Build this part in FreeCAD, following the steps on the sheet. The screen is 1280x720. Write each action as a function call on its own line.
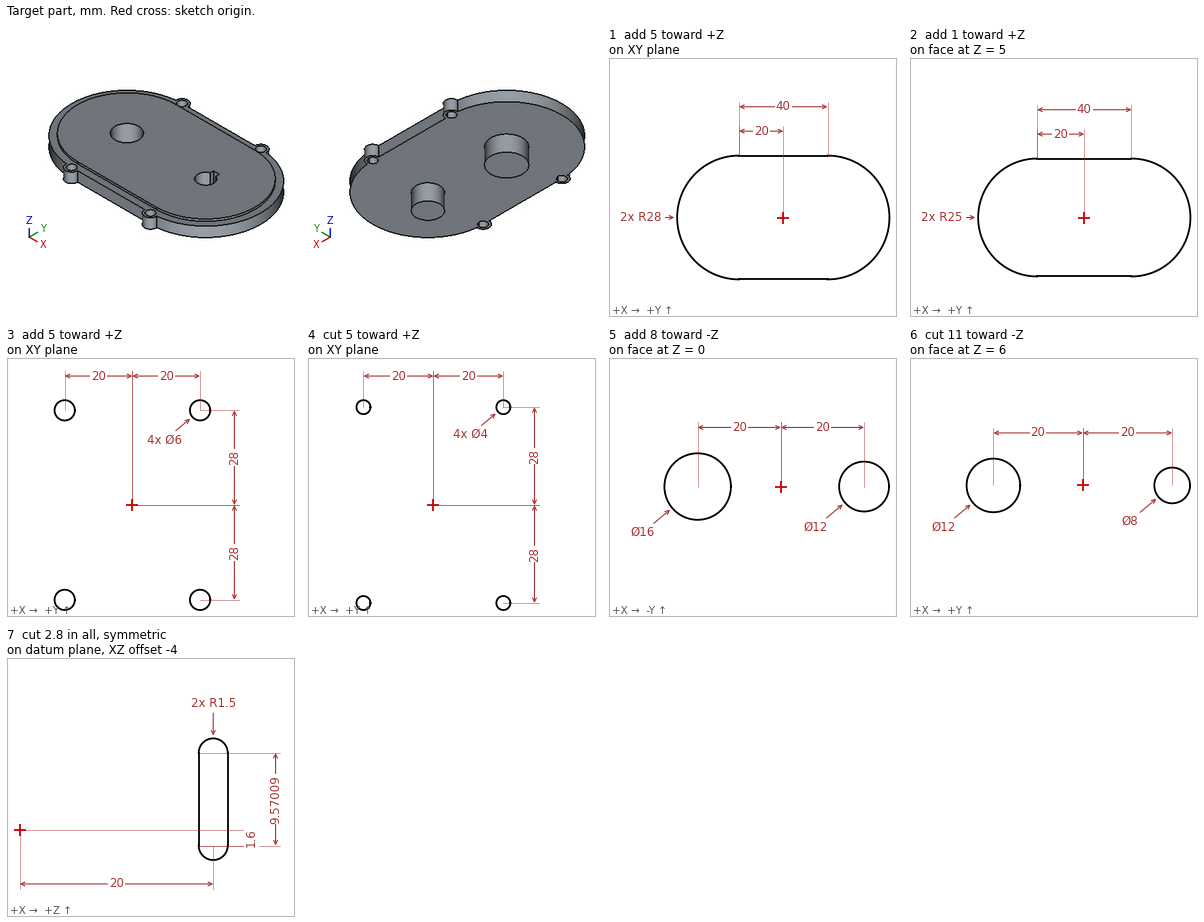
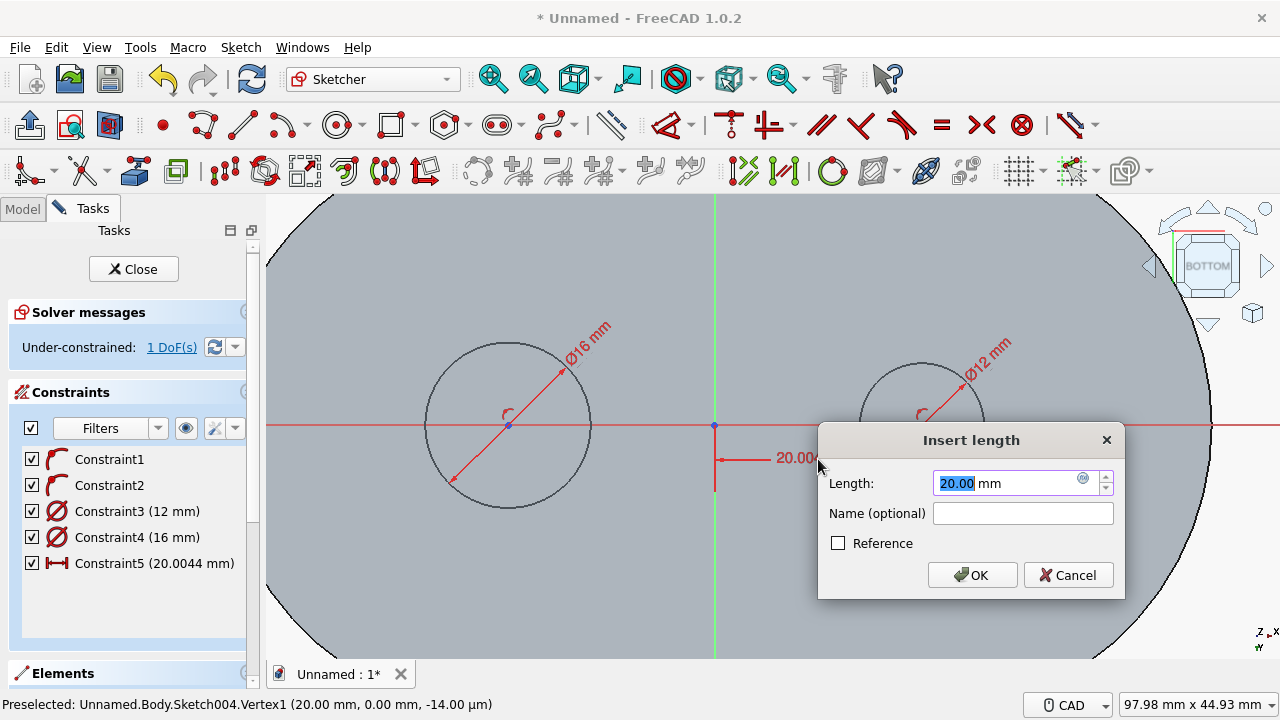
text(20)
key(Return)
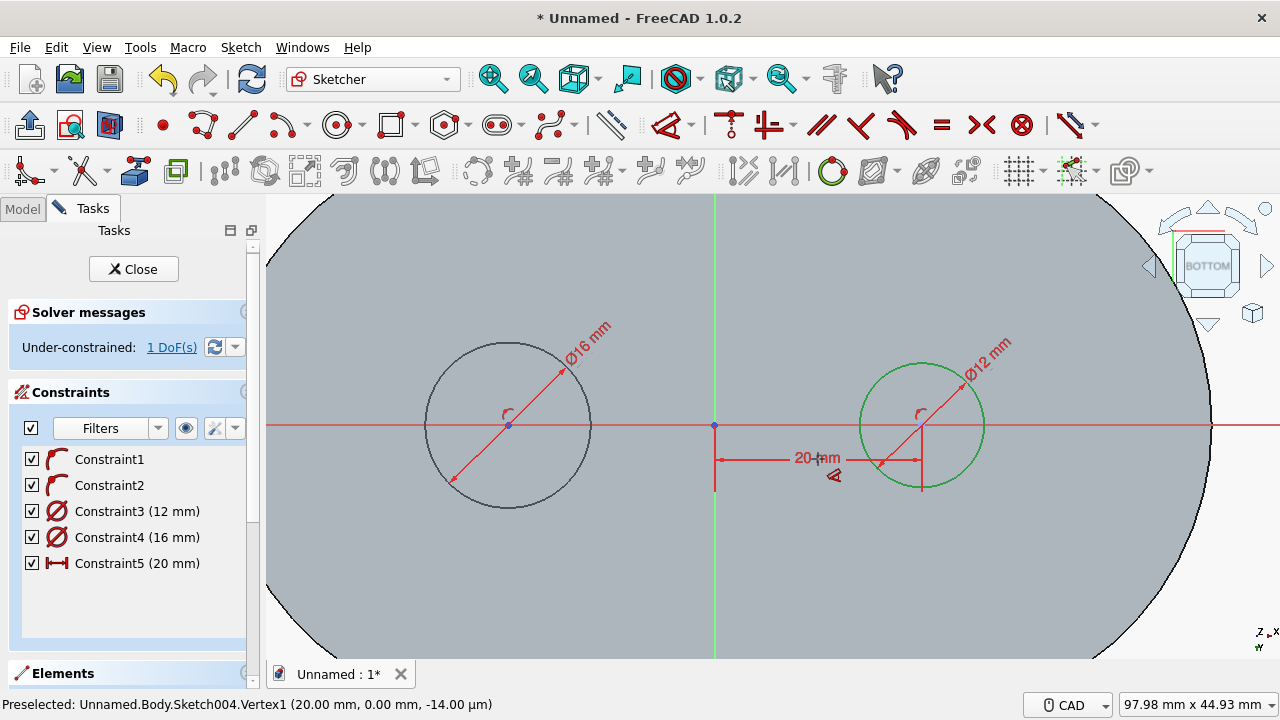
click(508, 425)
click(611, 459)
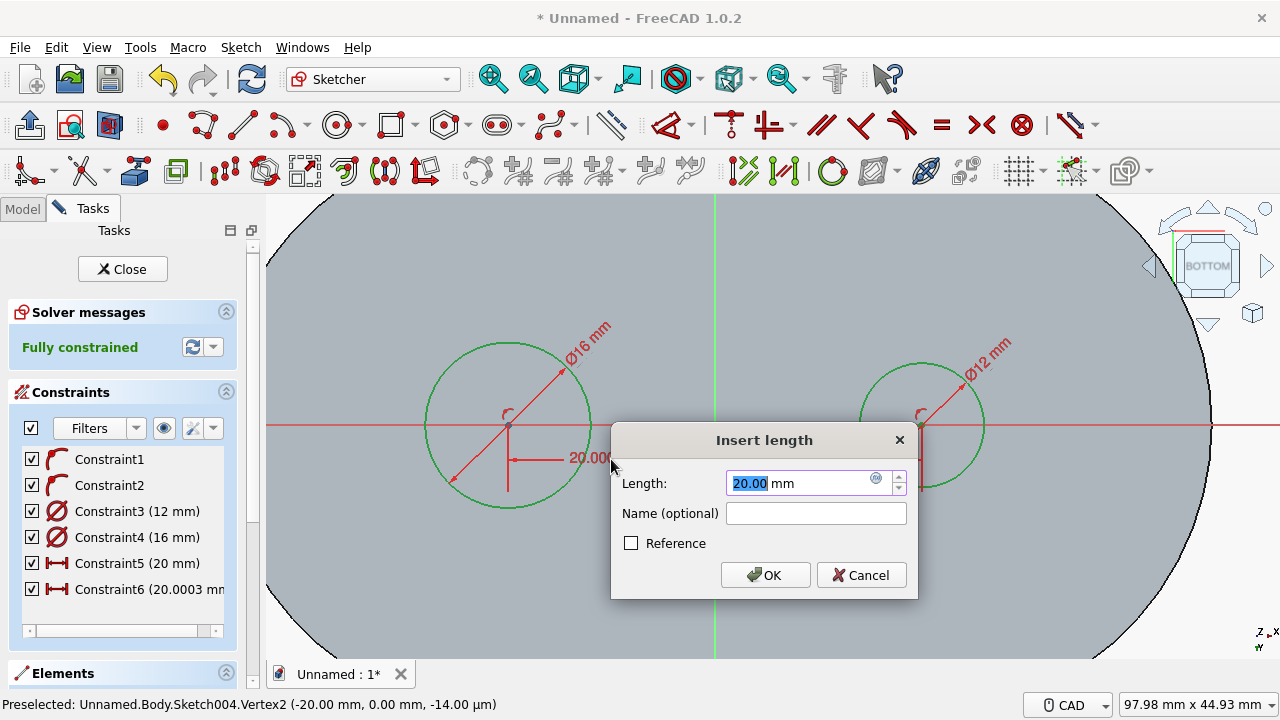
text(20)
key(Return)
key(Escape)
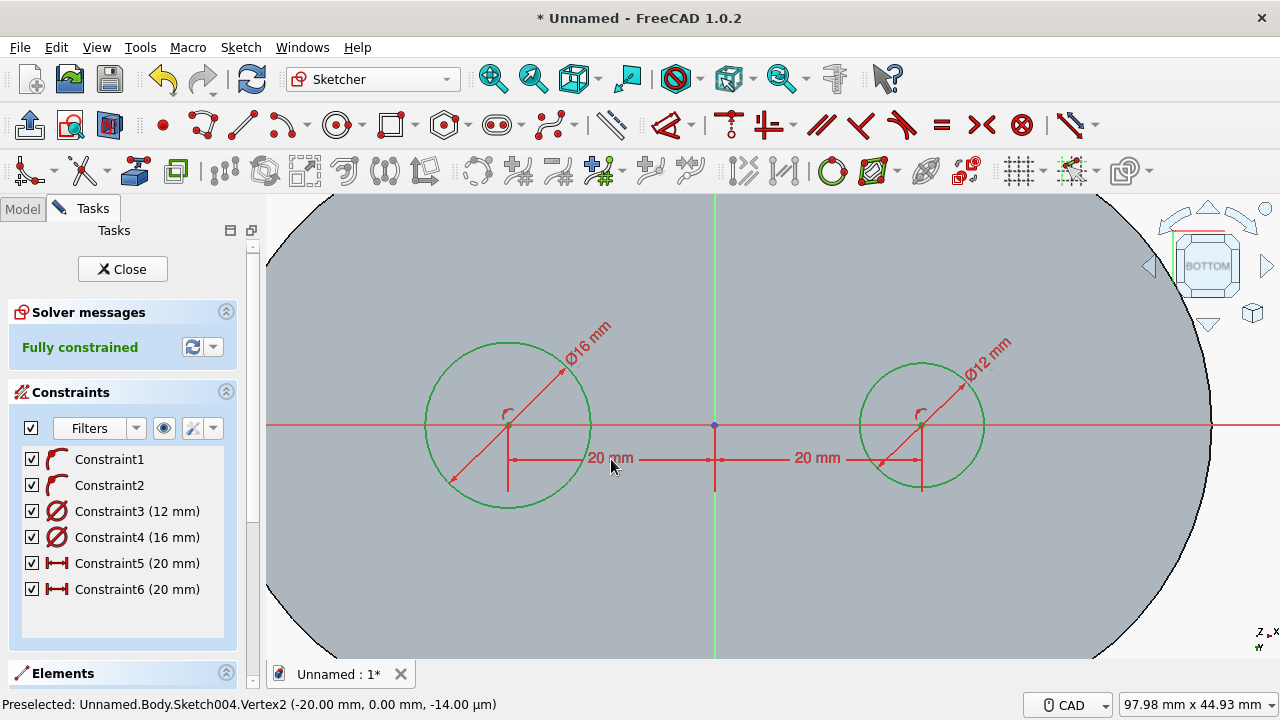
click(123, 269)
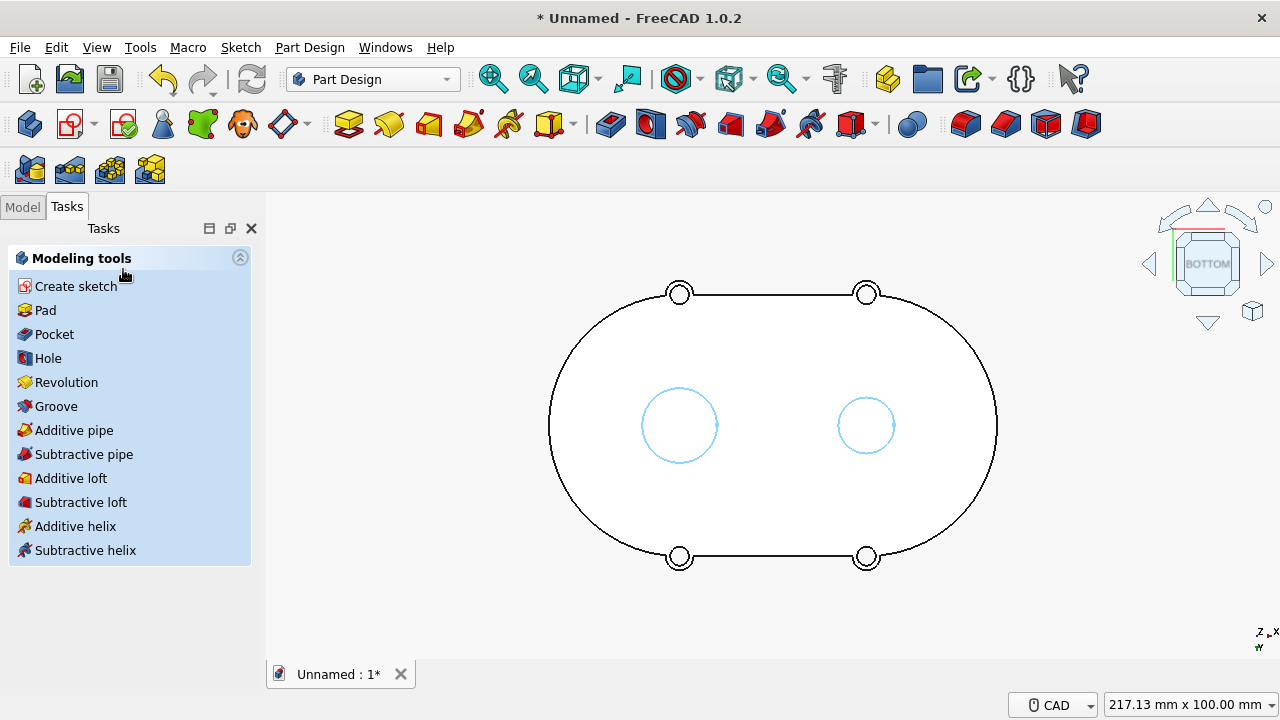
click(350, 124)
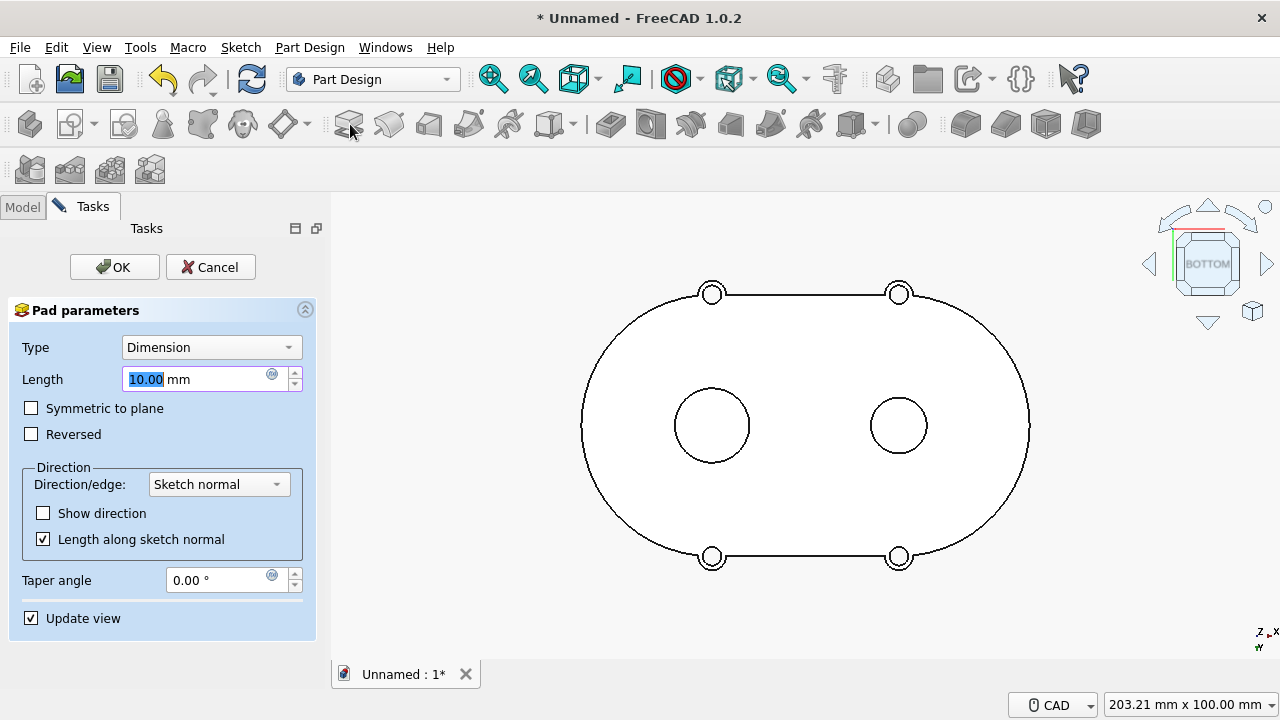
text(8)
key(Tab)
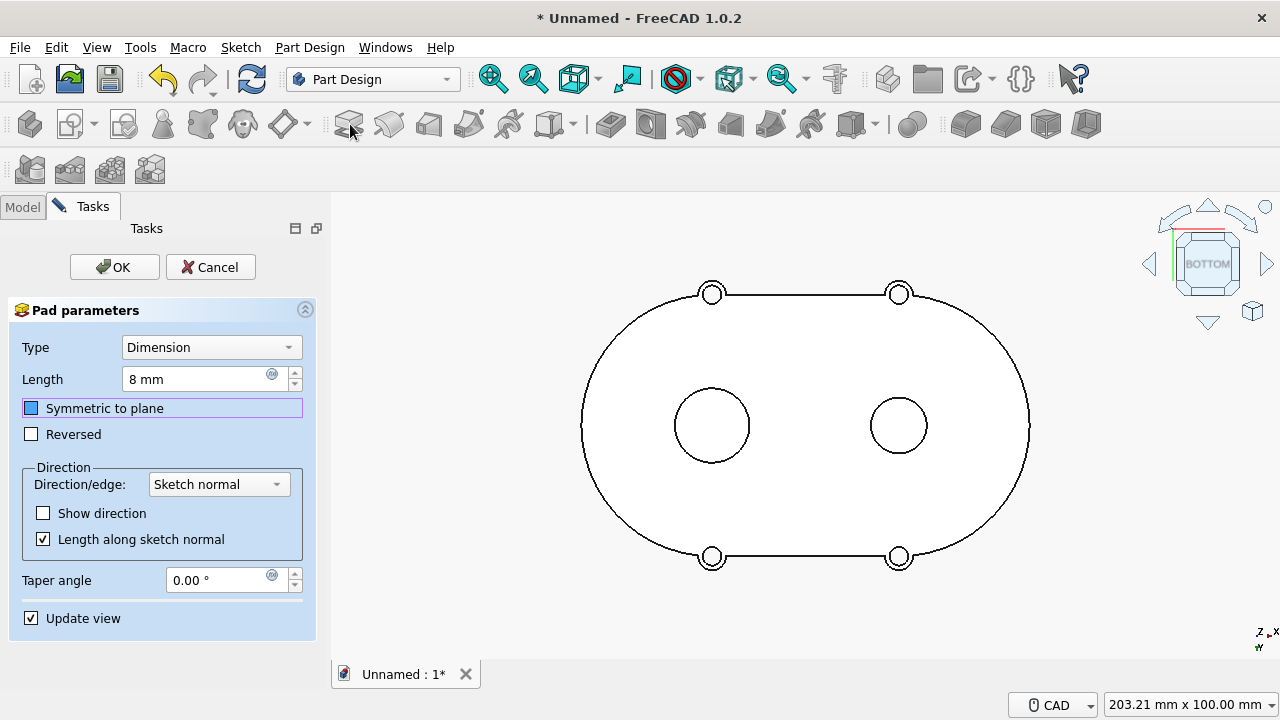
click(115, 267)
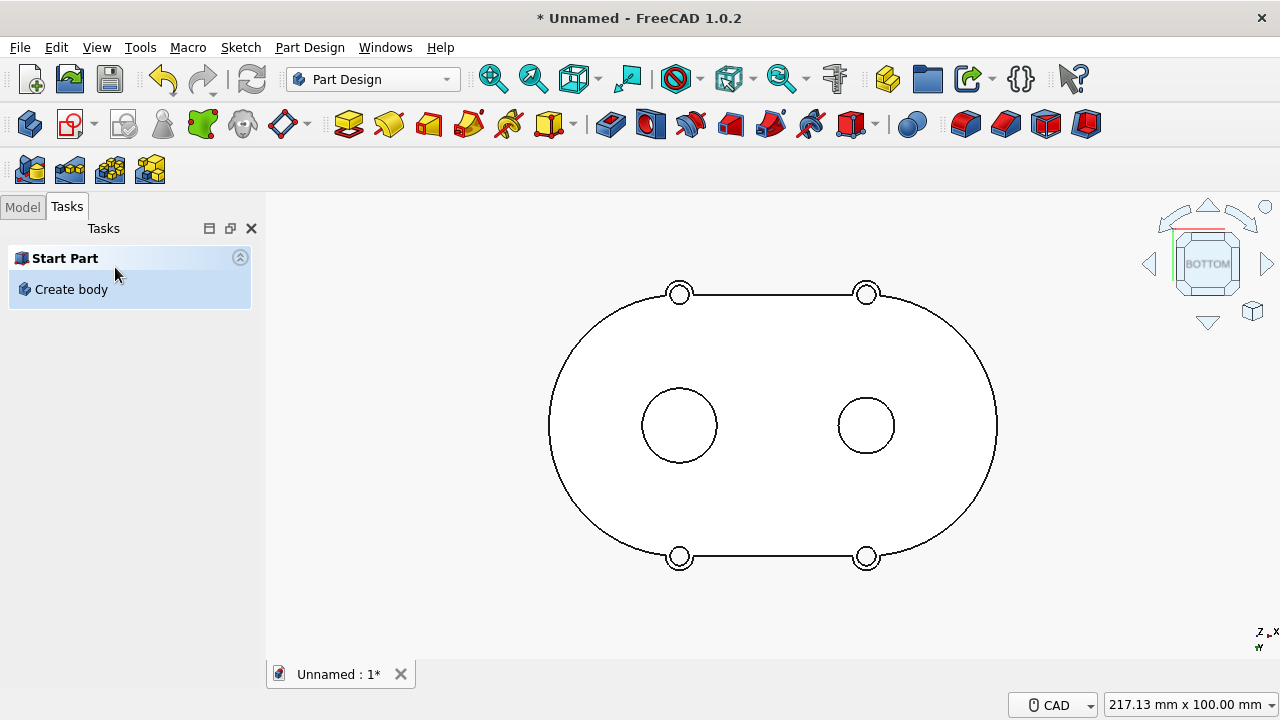
key(0)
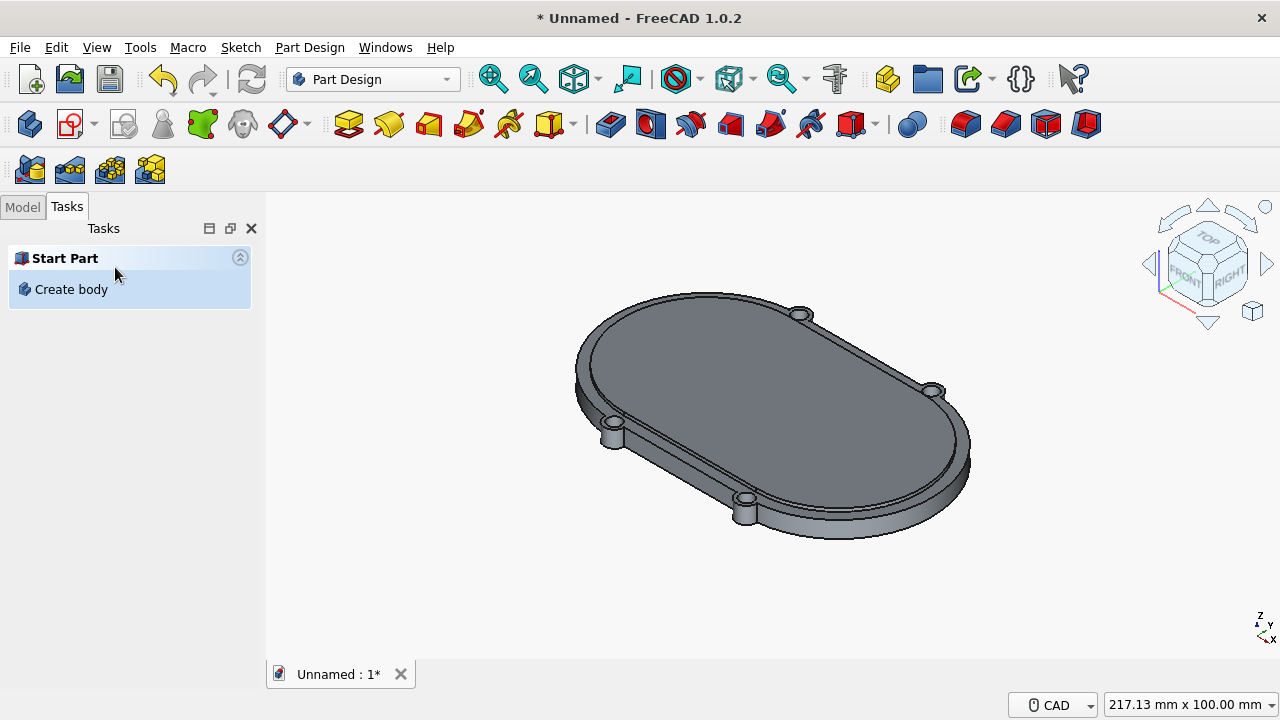
click(815, 426)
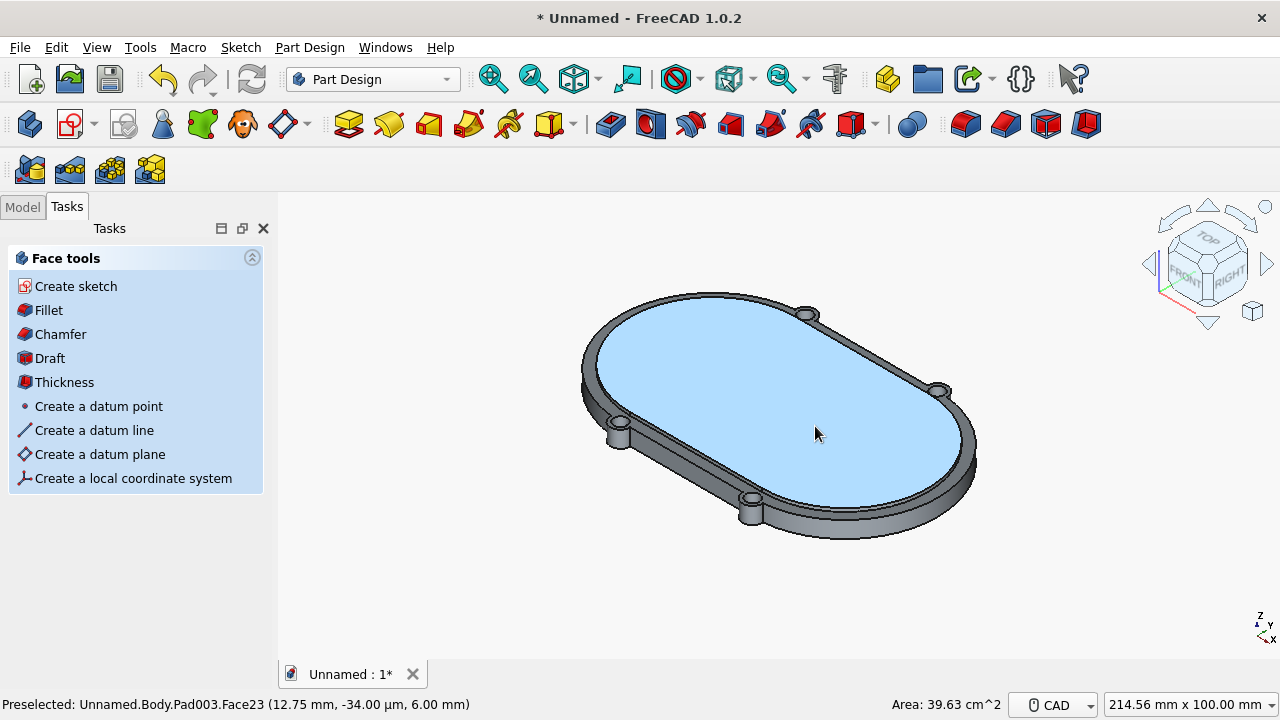
click(70, 124)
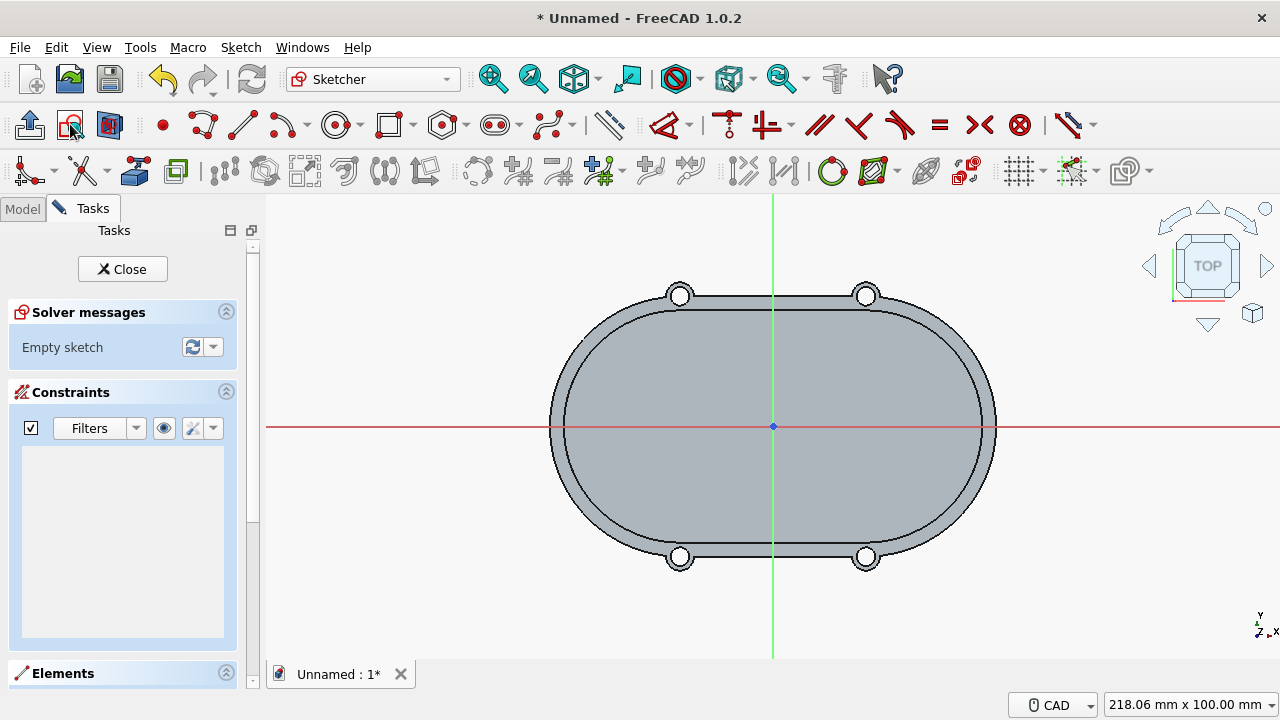
scroll(806, 426, up, 5)